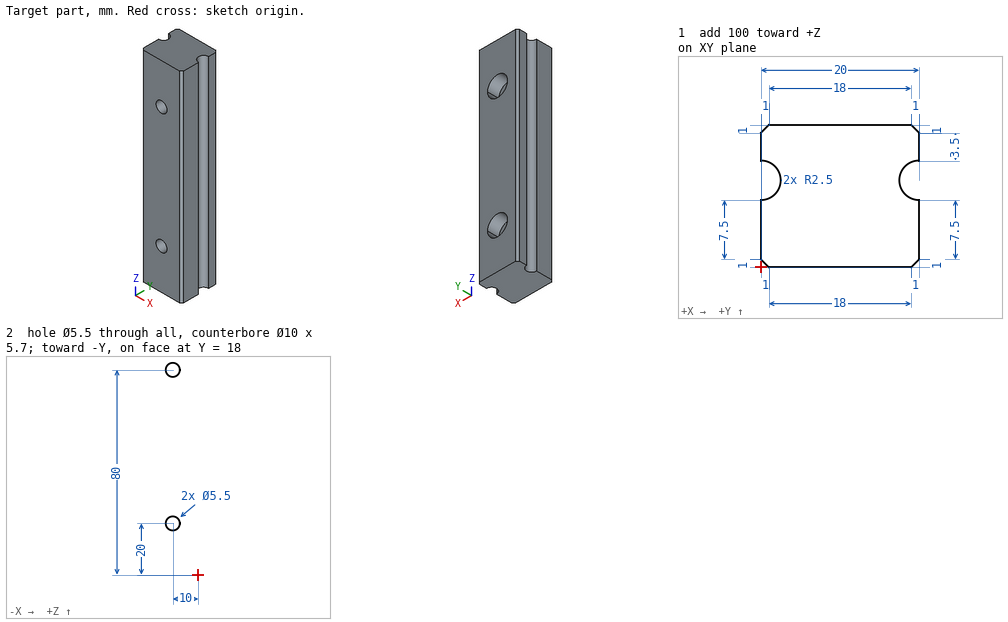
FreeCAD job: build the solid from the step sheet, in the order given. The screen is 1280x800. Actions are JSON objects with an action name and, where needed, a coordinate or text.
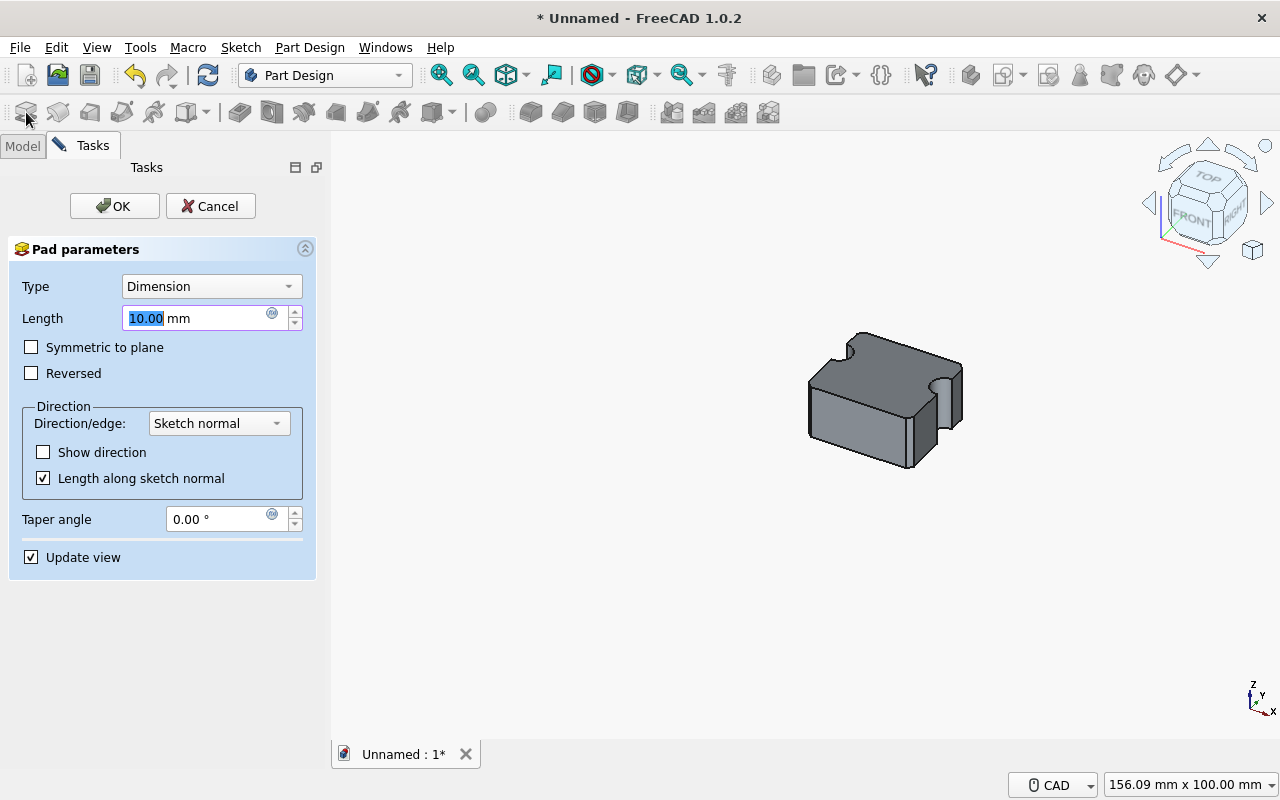
{"action": "type", "text": "100"}
{"action": "key", "text": "Tab"}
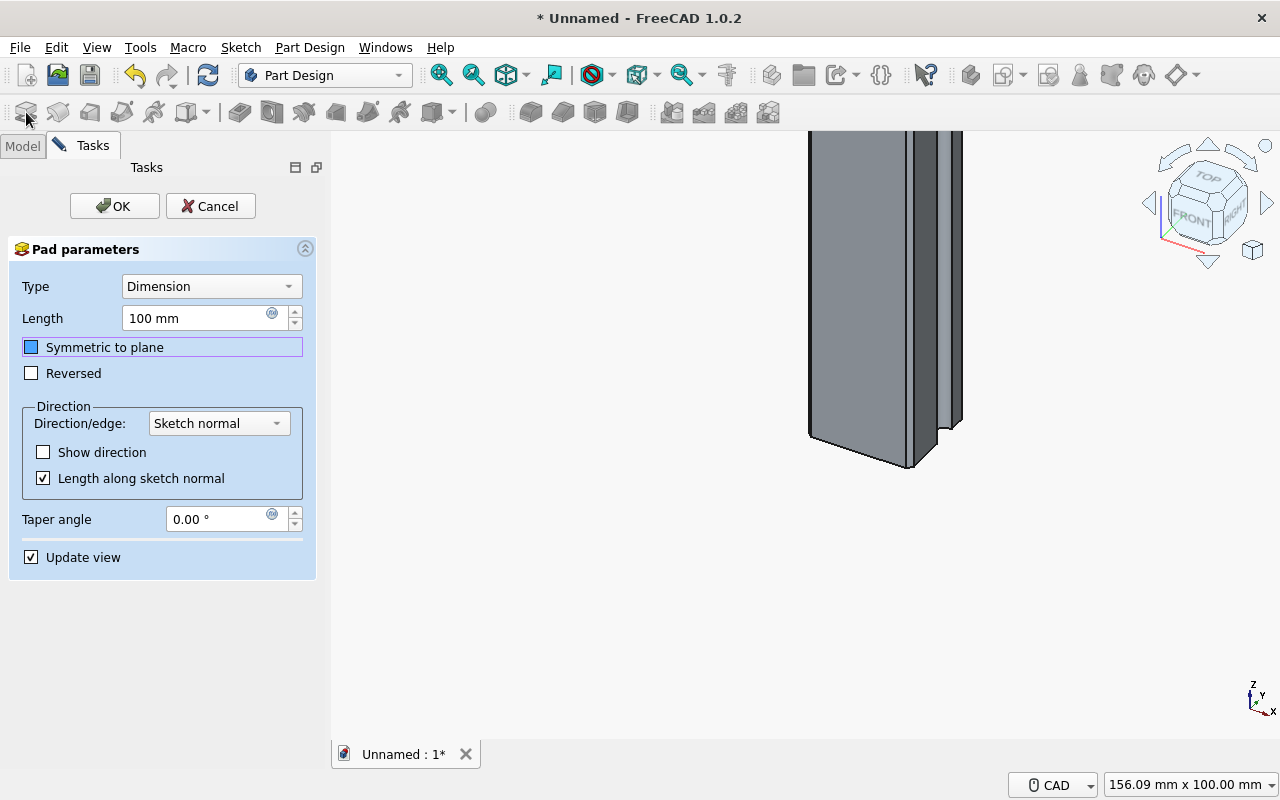
{"action": "left_click", "coordinate": [115, 206]}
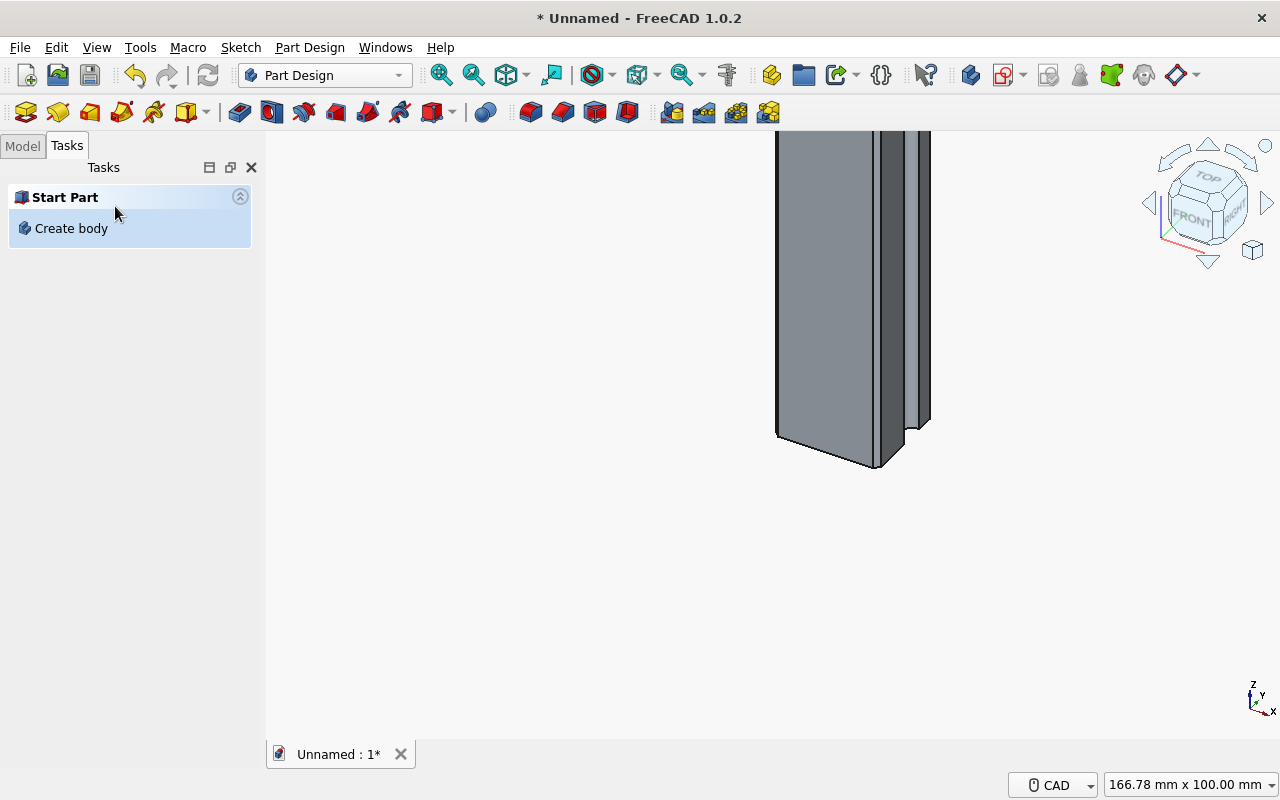
{"action": "left_click", "coordinate": [442, 76]}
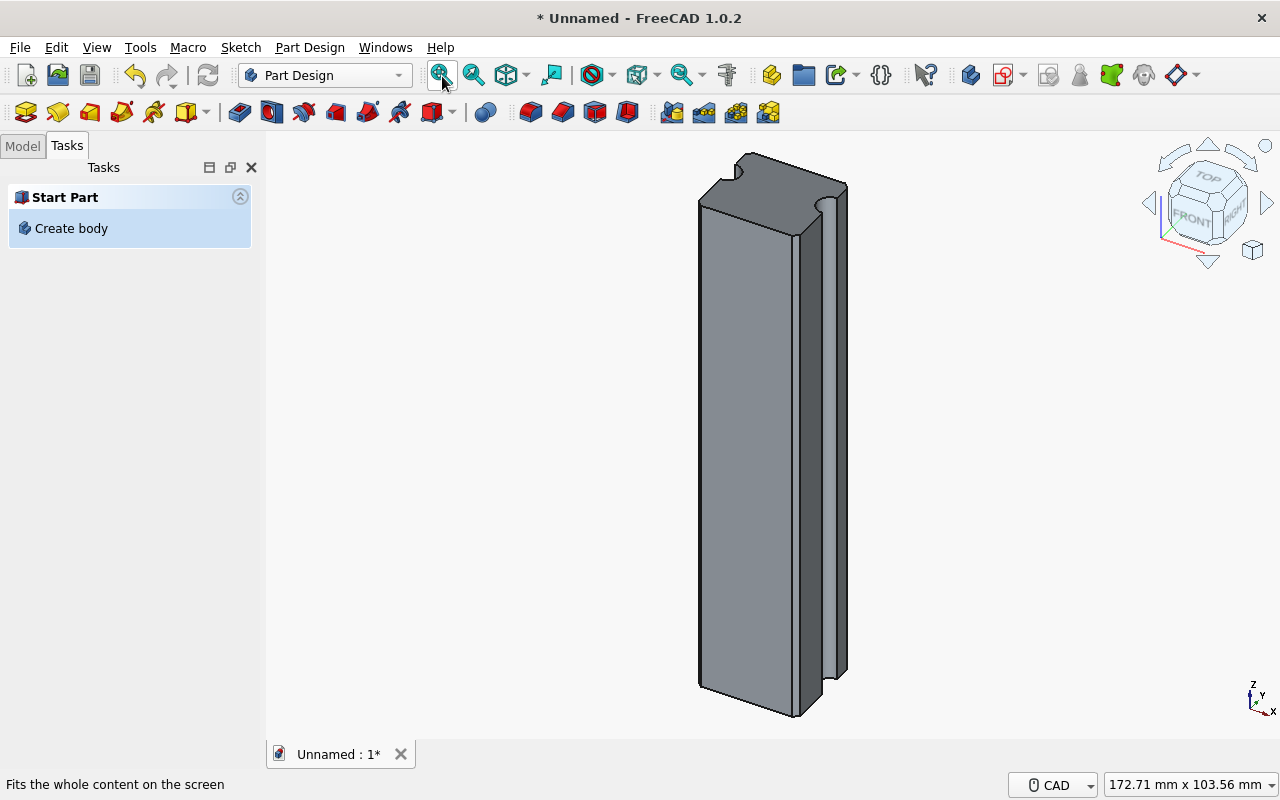
{"action": "key", "text": "4"}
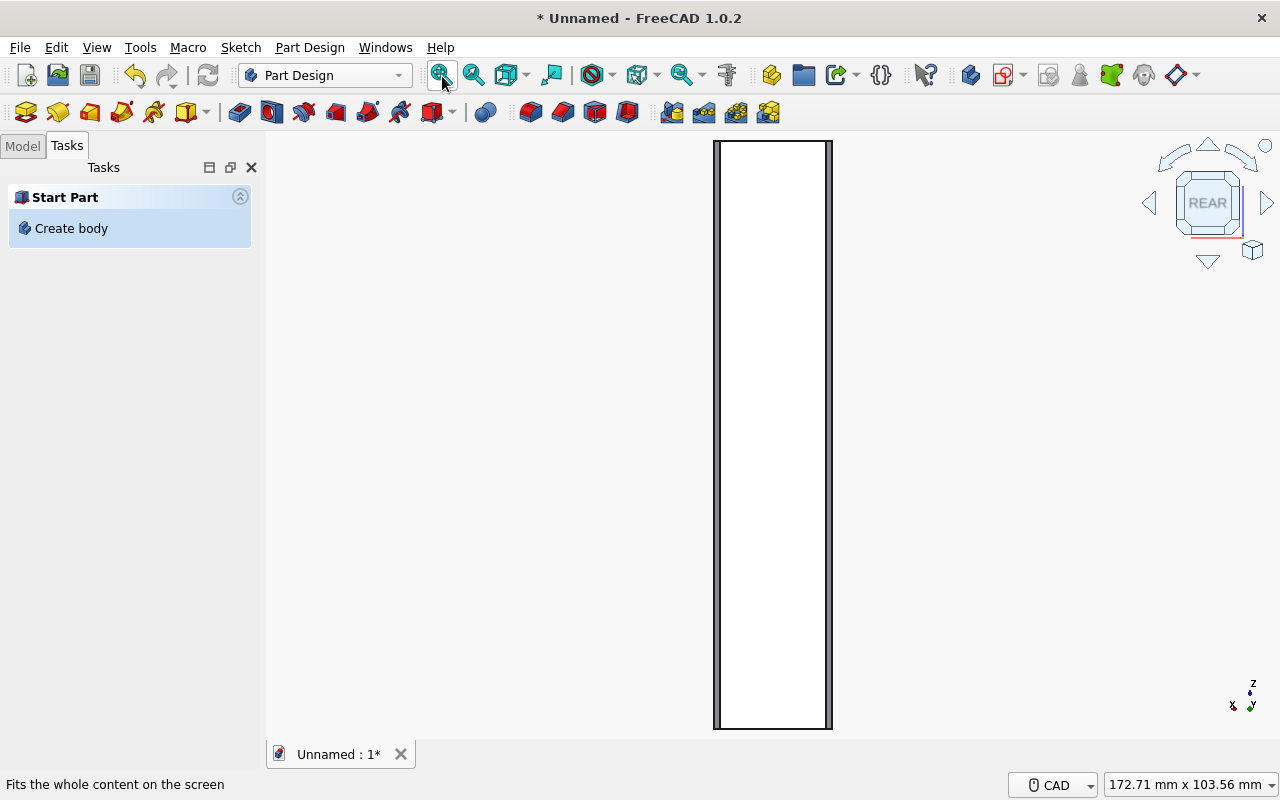
{"action": "left_click", "coordinate": [773, 266]}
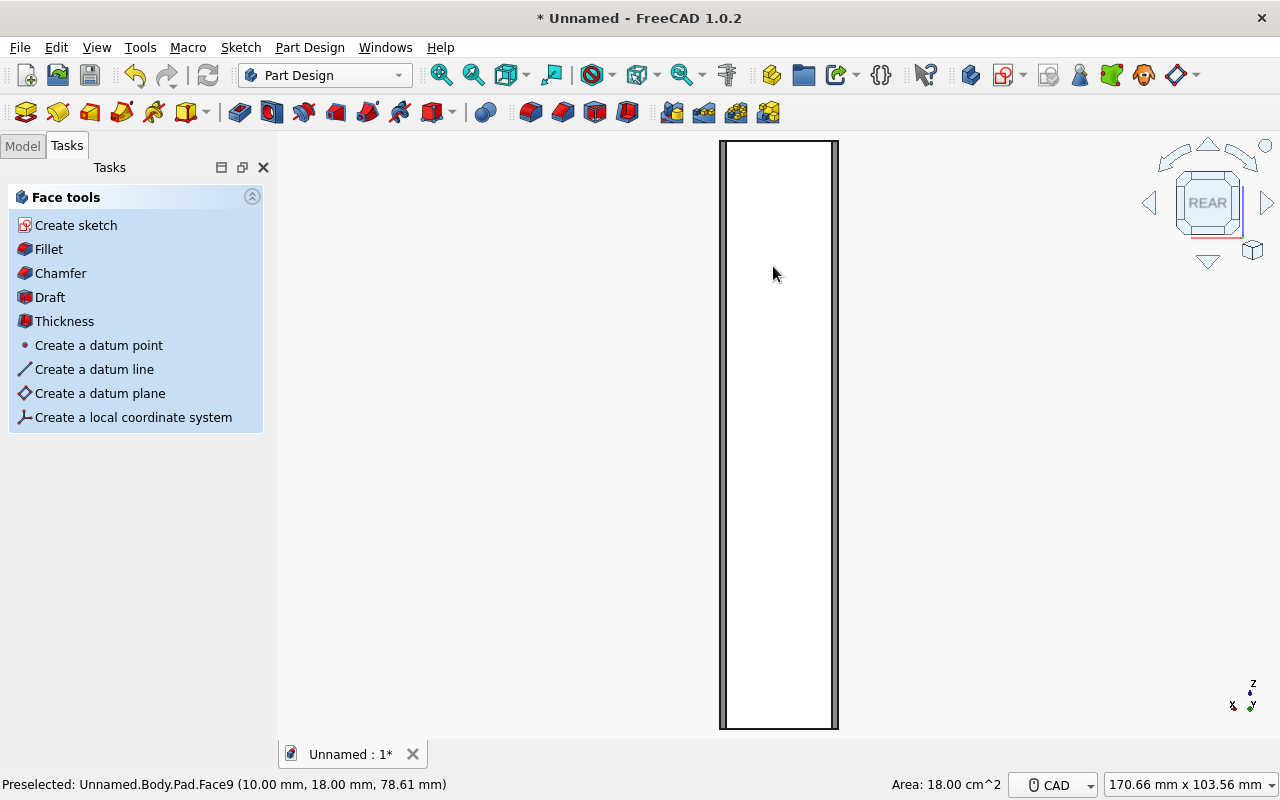
{"action": "left_click", "coordinate": [1004, 76]}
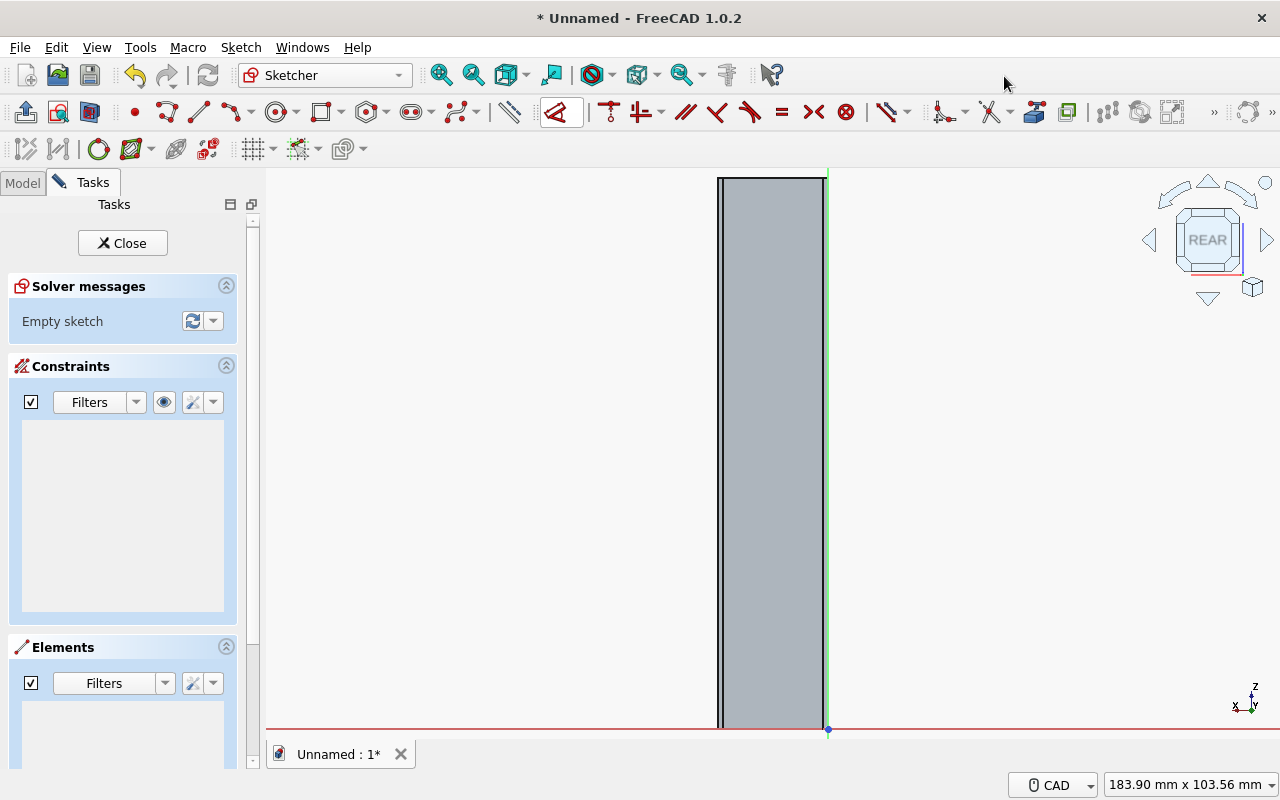
{"action": "scroll", "coordinate": [305, 239], "scroll_direction": "down", "scroll_amount": 1}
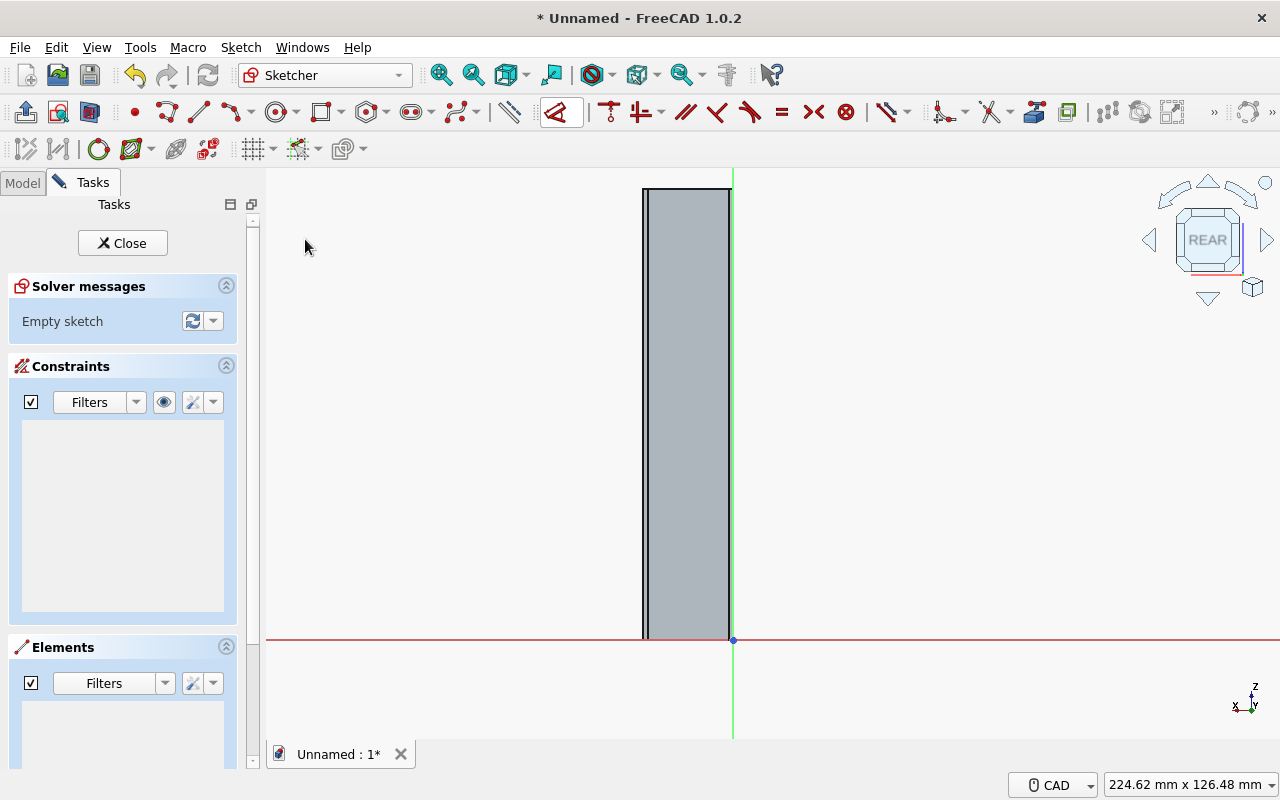
{"action": "left_click", "coordinate": [276, 112]}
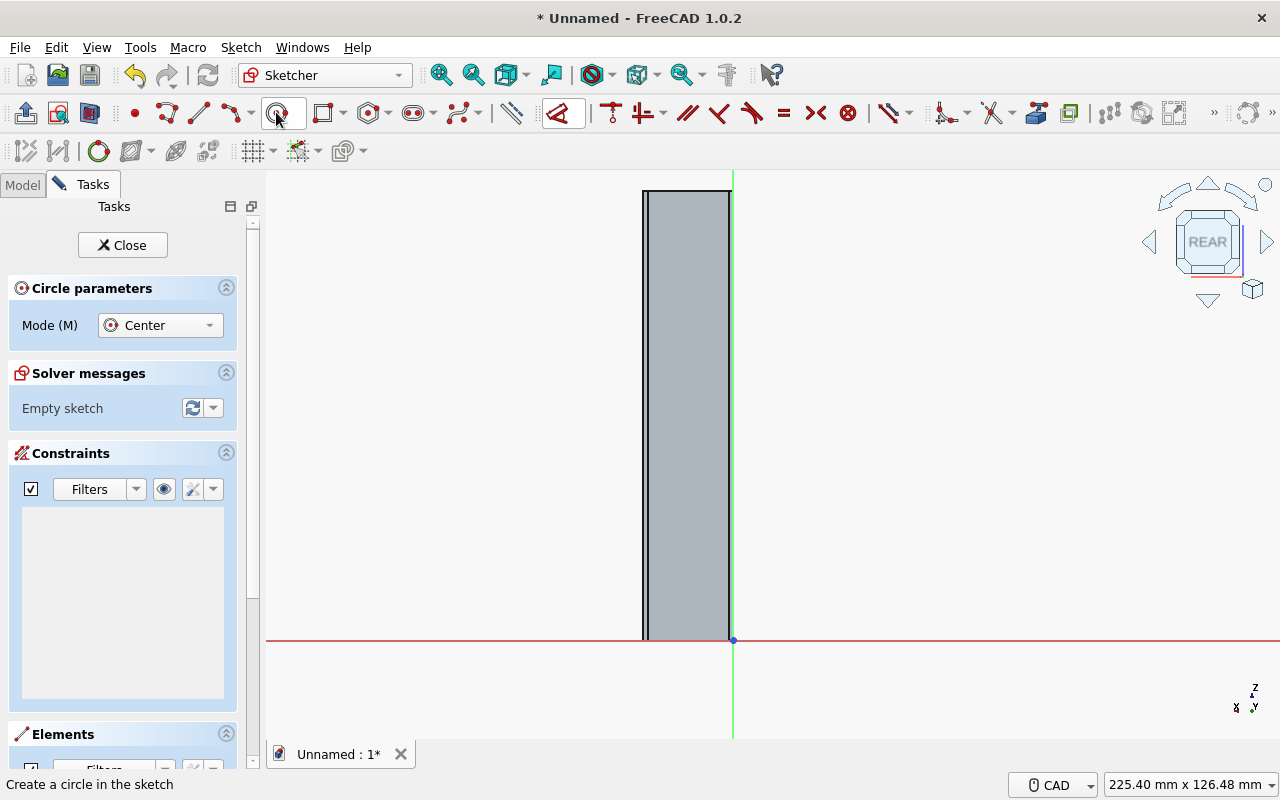
{"action": "scroll", "coordinate": [688, 551], "scroll_direction": "up", "scroll_amount": 4}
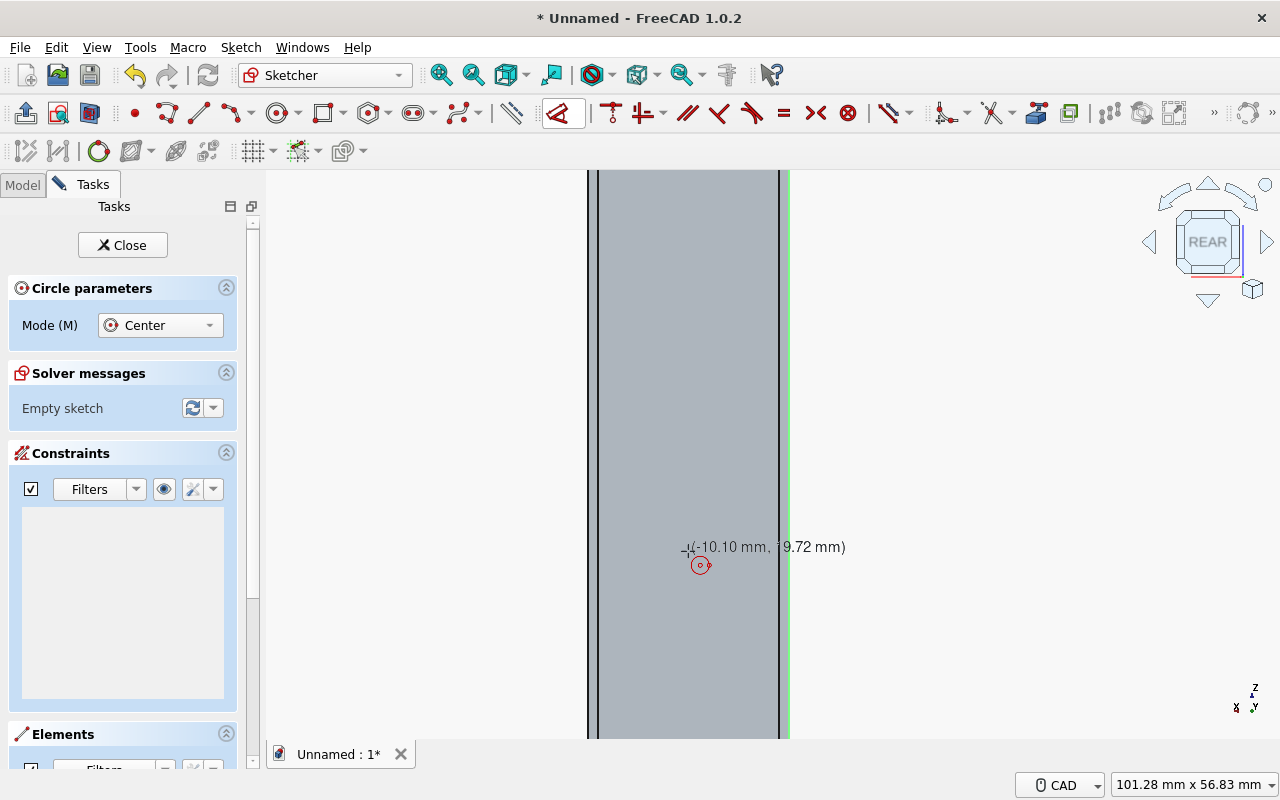
{"action": "left_click", "coordinate": [689, 550]}
{"action": "mouse_move", "coordinate": [708, 530]}